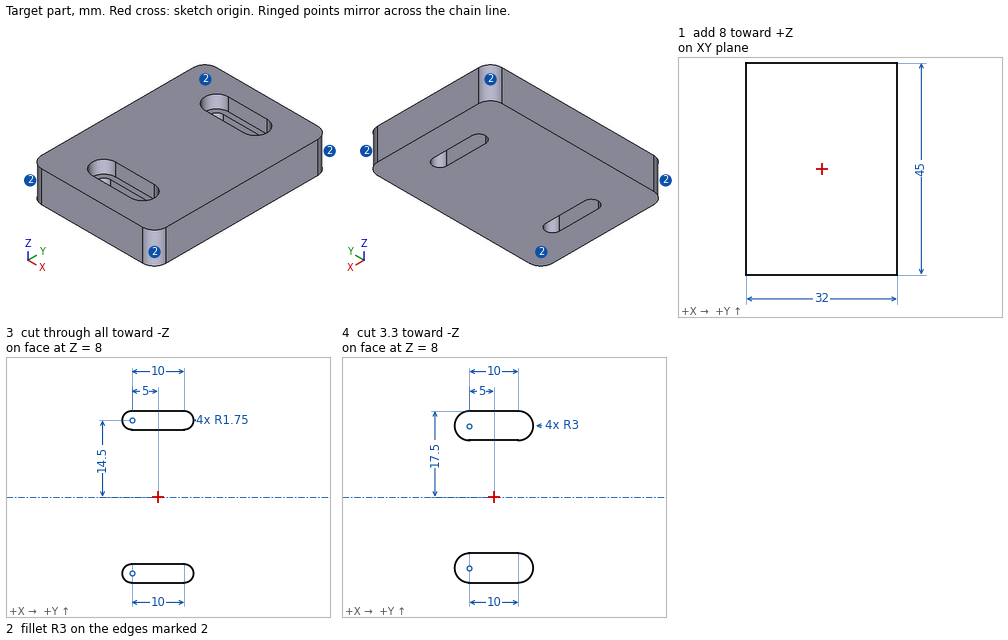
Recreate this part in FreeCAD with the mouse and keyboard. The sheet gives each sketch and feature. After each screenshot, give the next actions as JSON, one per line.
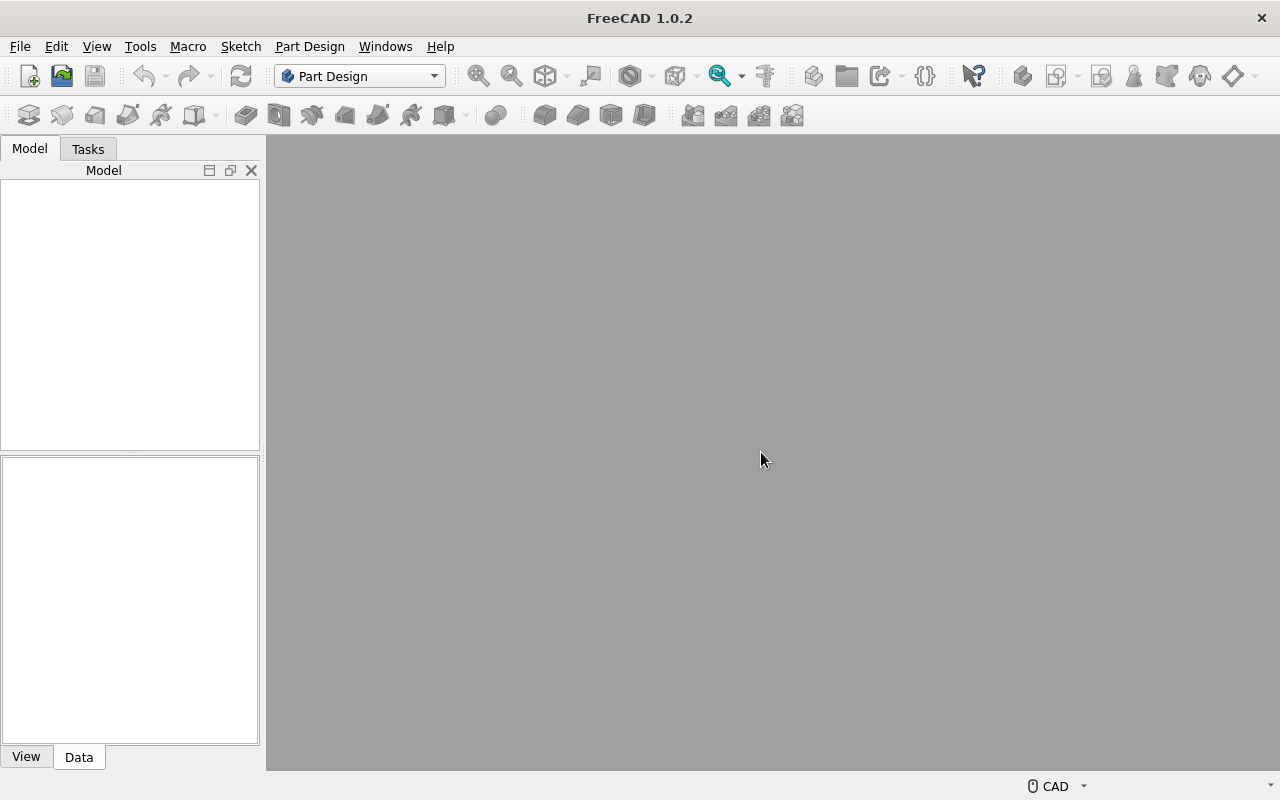
{"action": "left_click", "coordinate": [29, 76]}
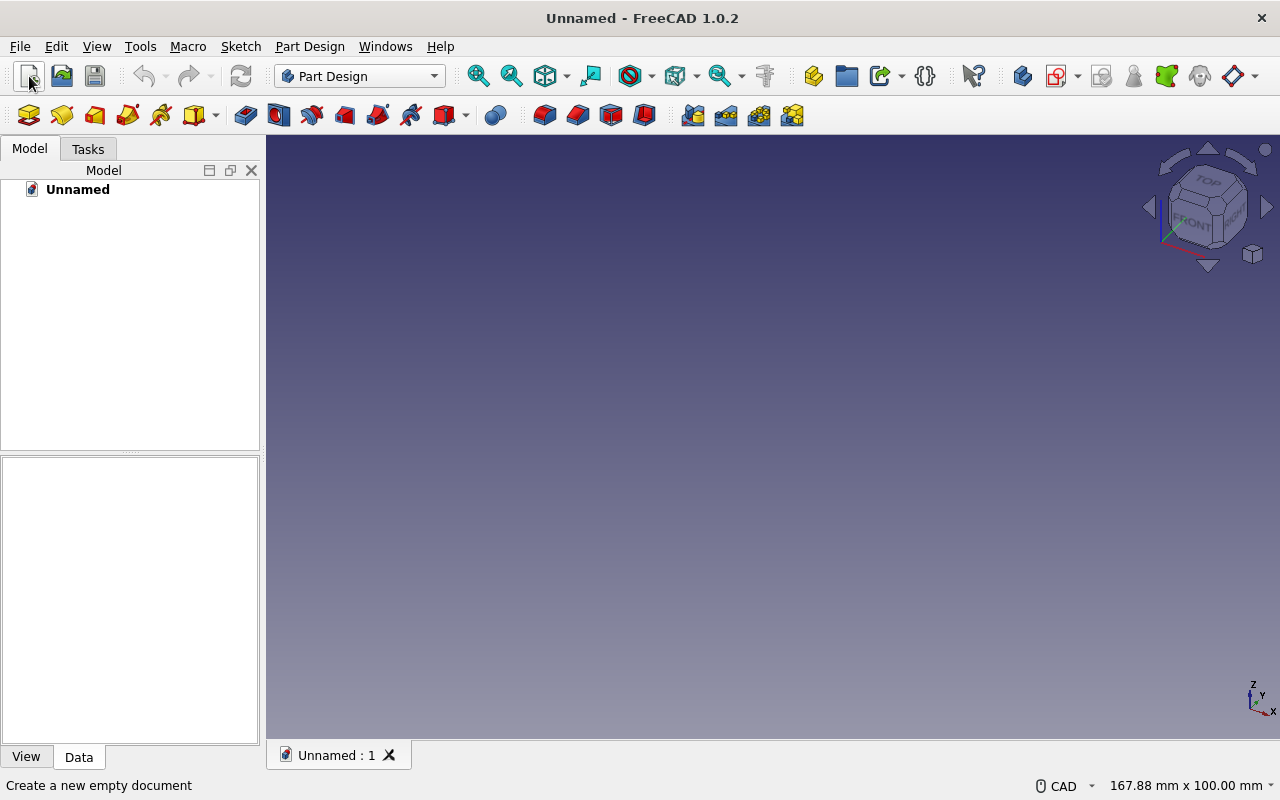
{"action": "left_click", "coordinate": [1056, 76]}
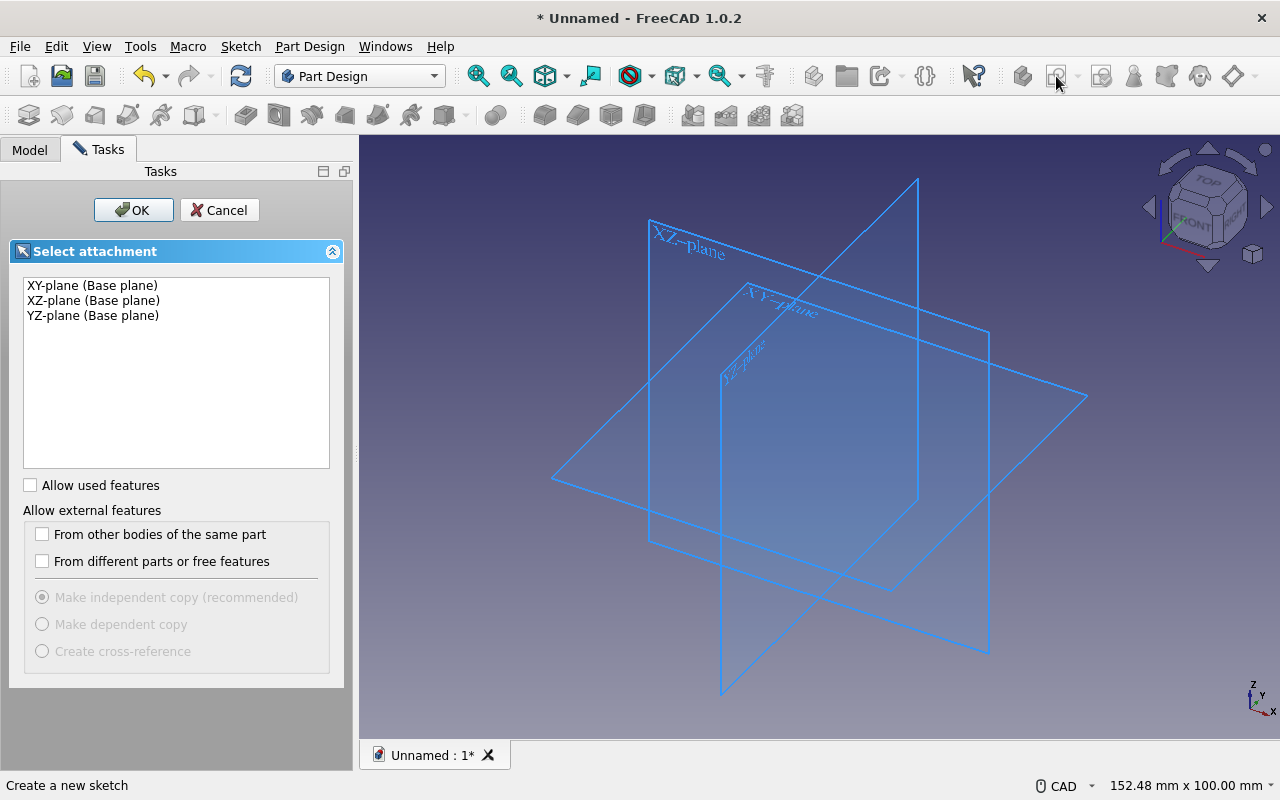
{"action": "left_click", "coordinate": [84, 286]}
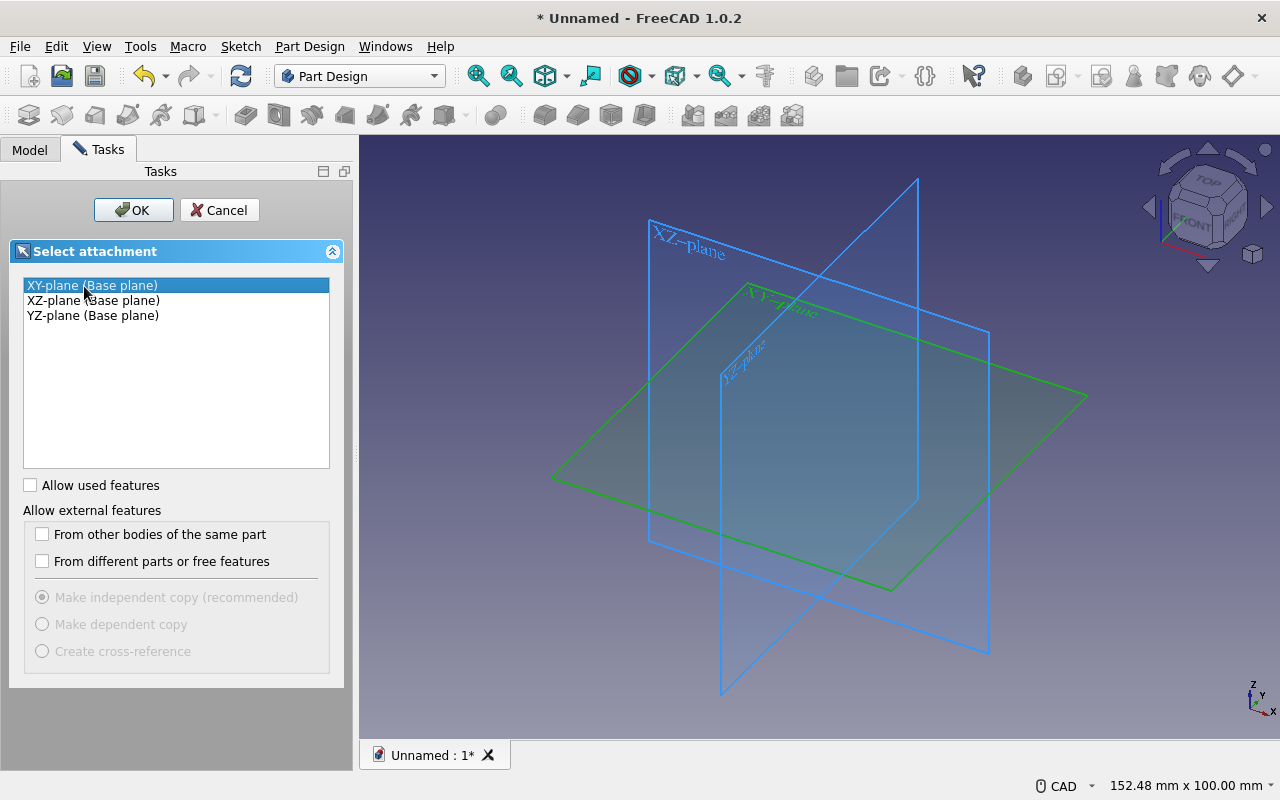
{"action": "left_click", "coordinate": [134, 210]}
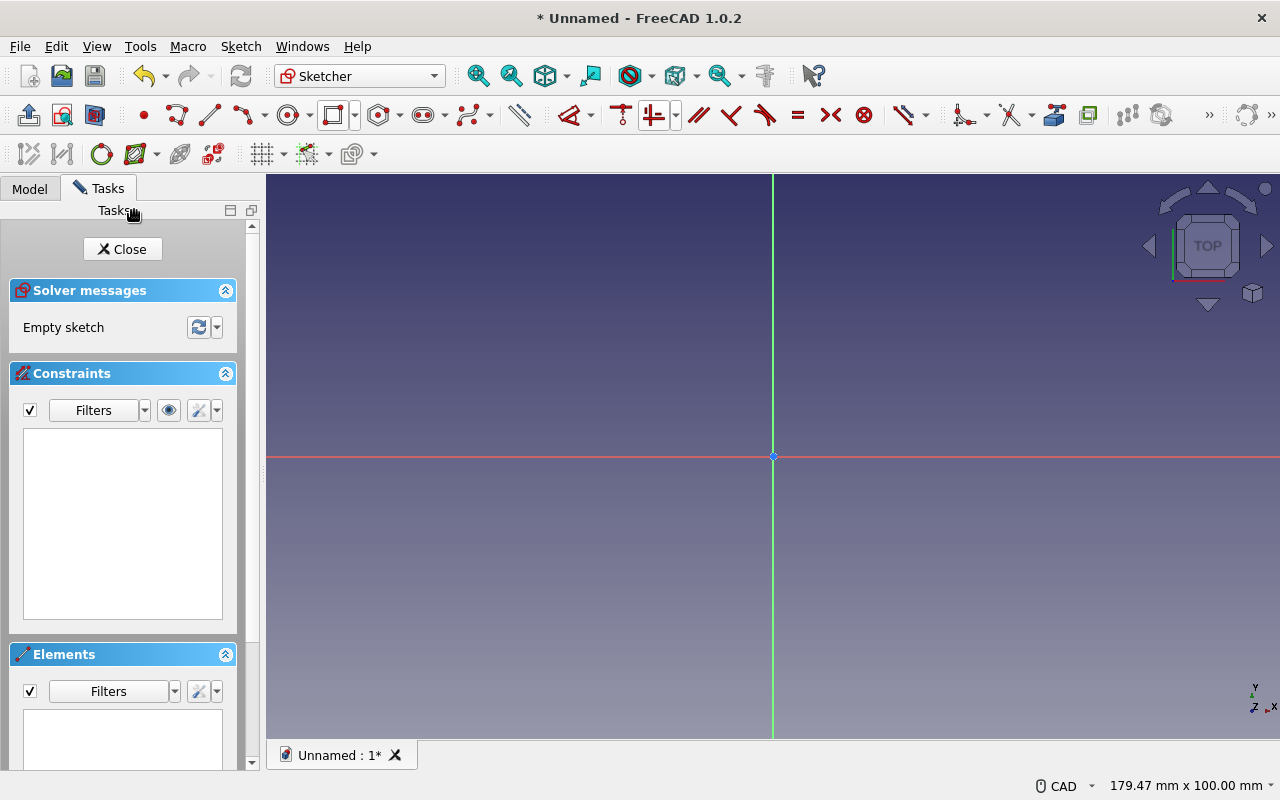
{"action": "scroll", "coordinate": [912, 456], "scroll_direction": "up", "scroll_amount": 2}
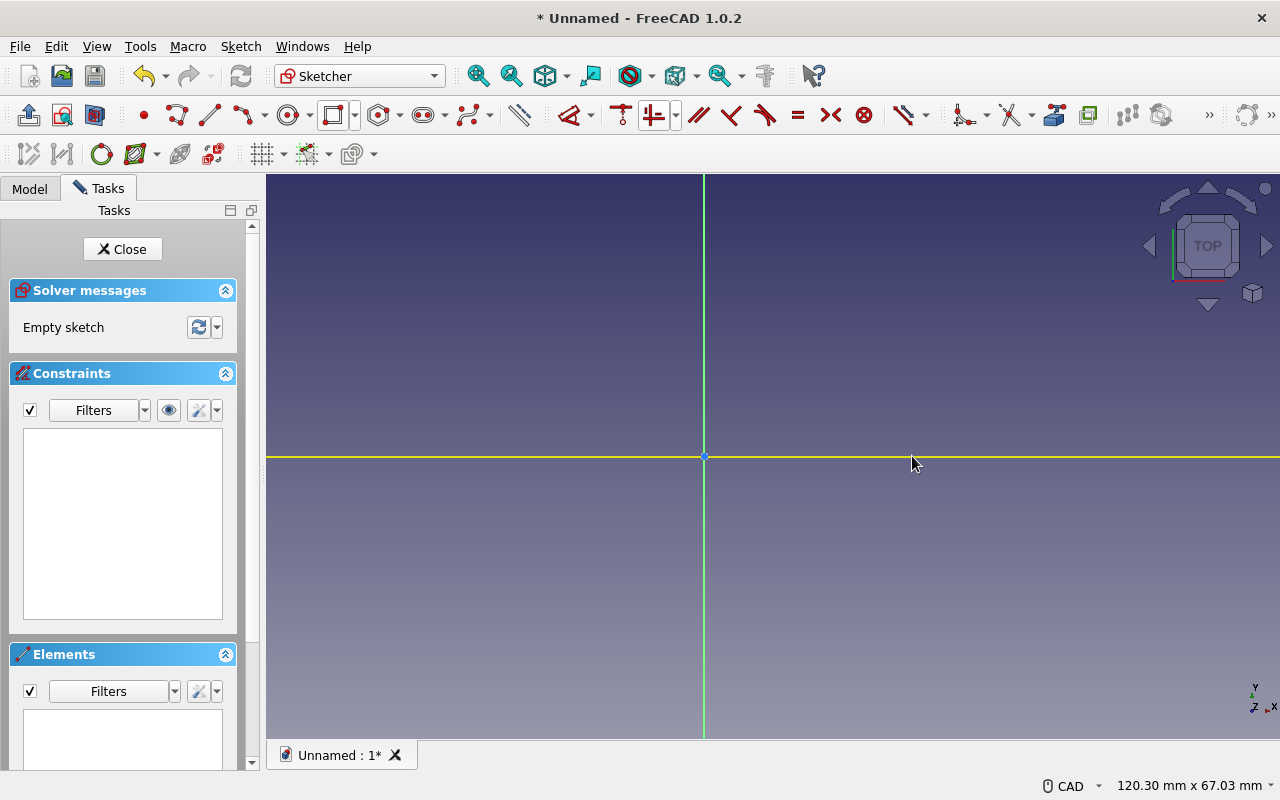
{"action": "left_click", "coordinate": [354, 116]}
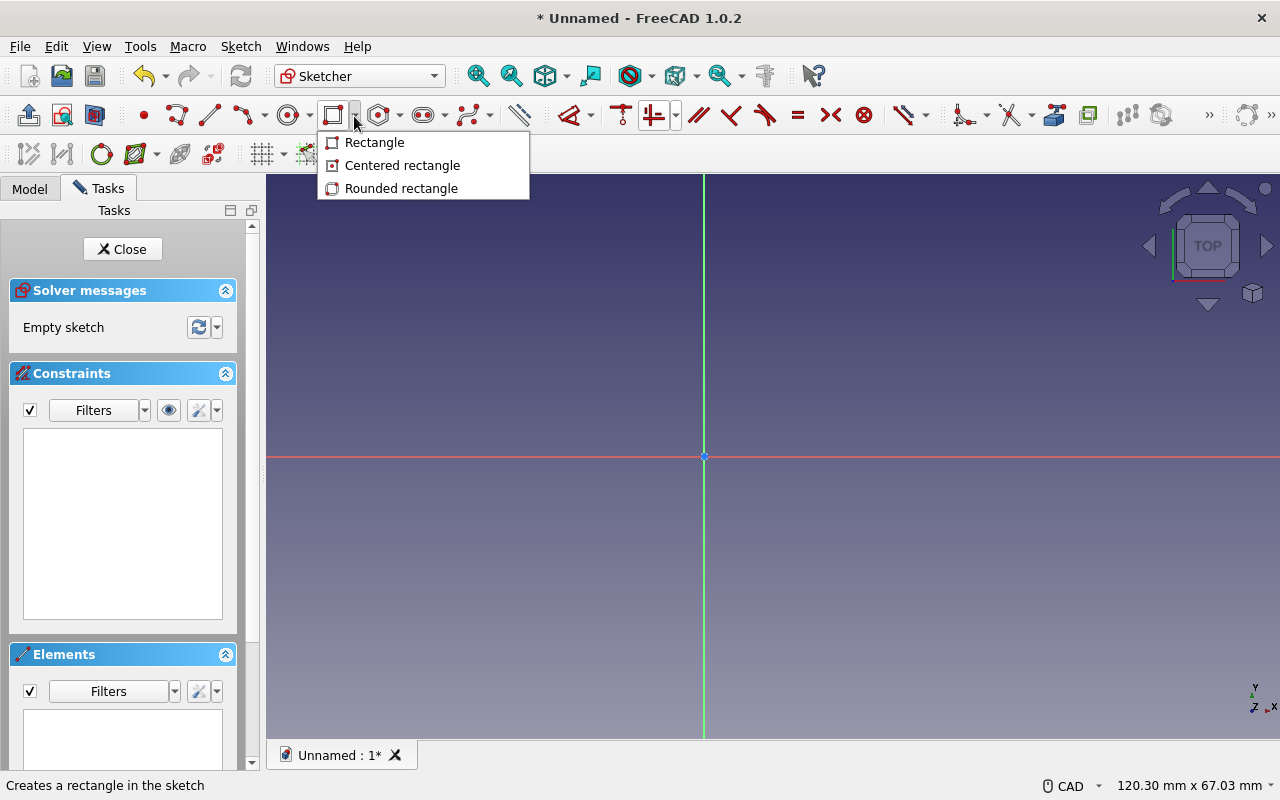
{"action": "left_click", "coordinate": [424, 166]}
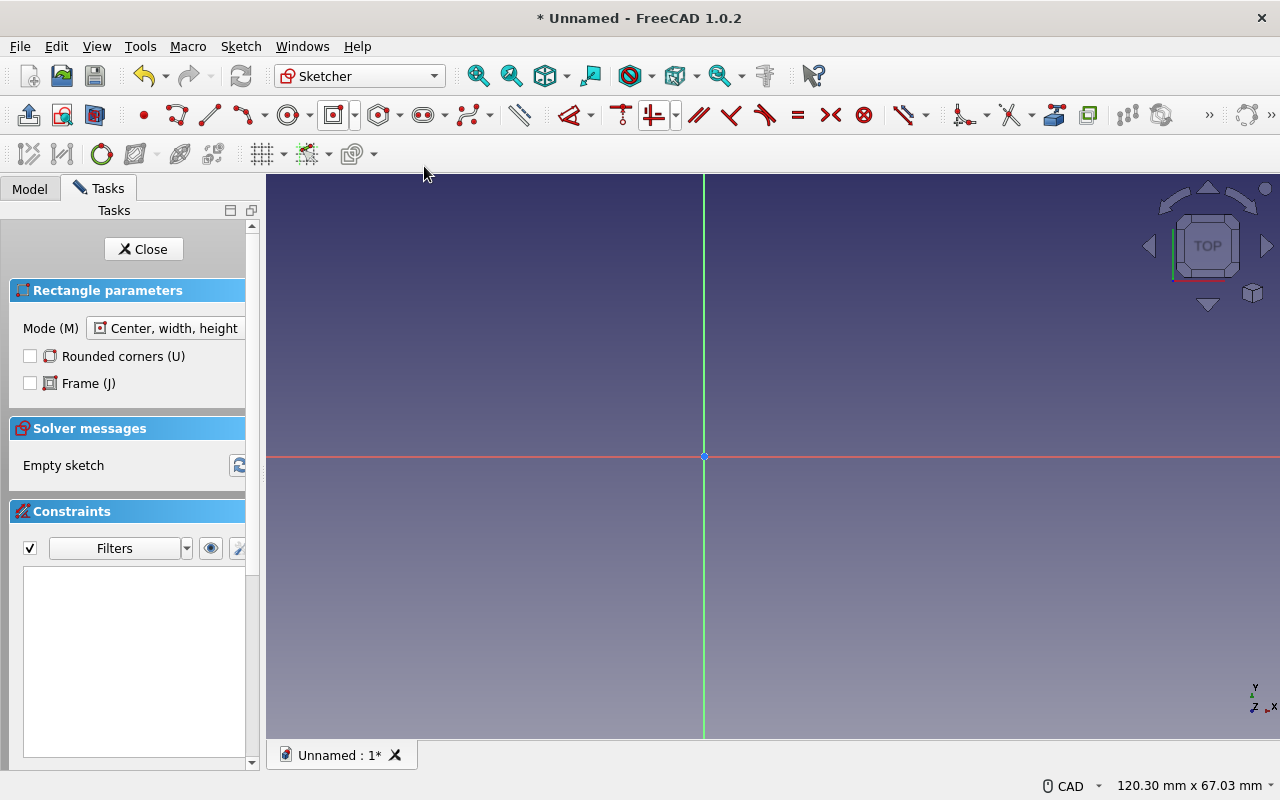
{"action": "left_click", "coordinate": [704, 456]}
{"action": "left_click", "coordinate": [839, 267]}
{"action": "key", "text": "Escape"}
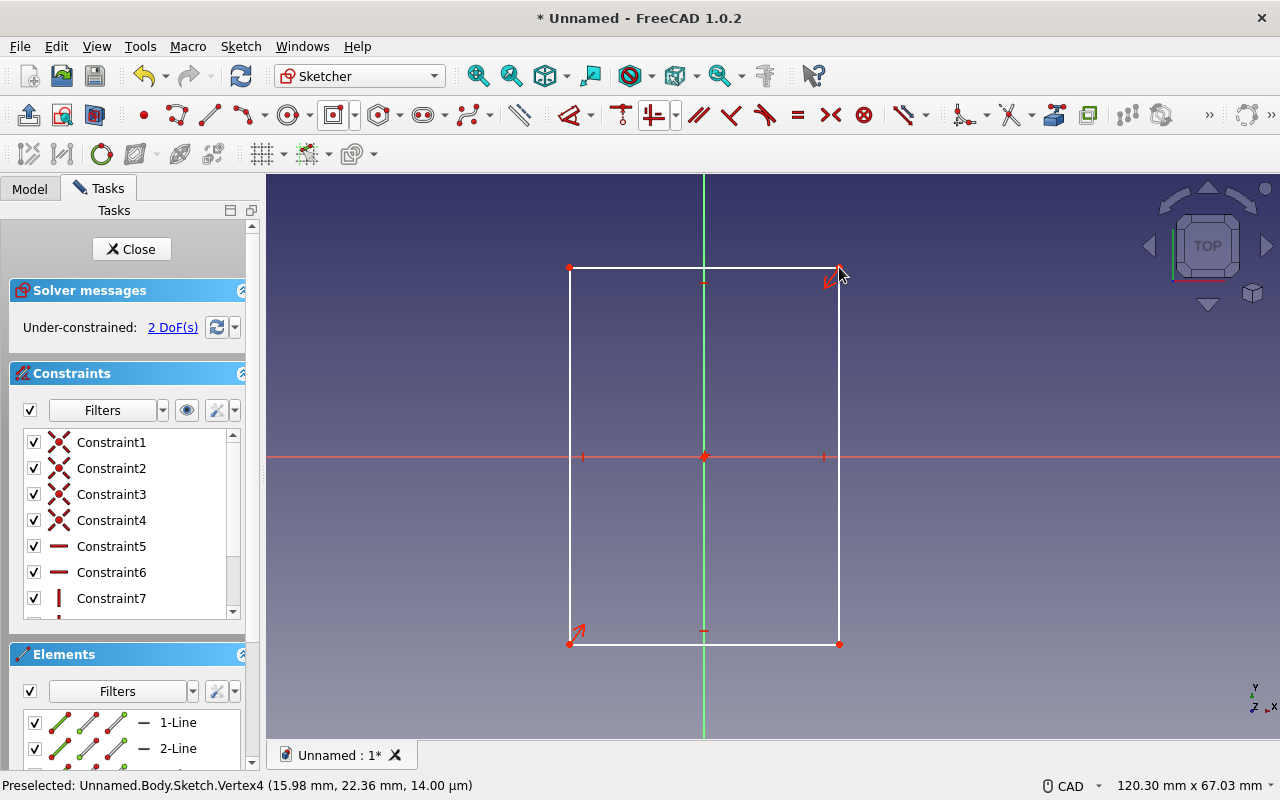
{"action": "left_click", "coordinate": [650, 645]}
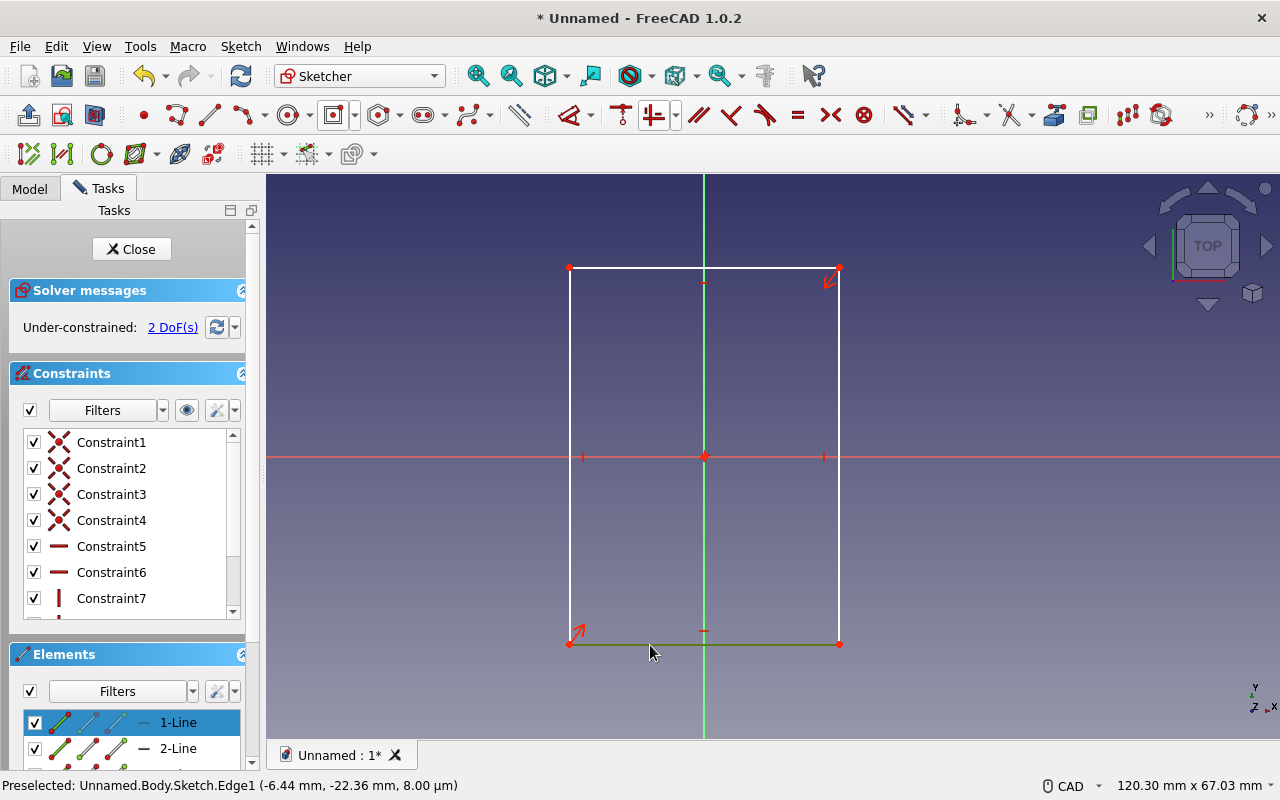
{"action": "left_click", "coordinate": [590, 116]}